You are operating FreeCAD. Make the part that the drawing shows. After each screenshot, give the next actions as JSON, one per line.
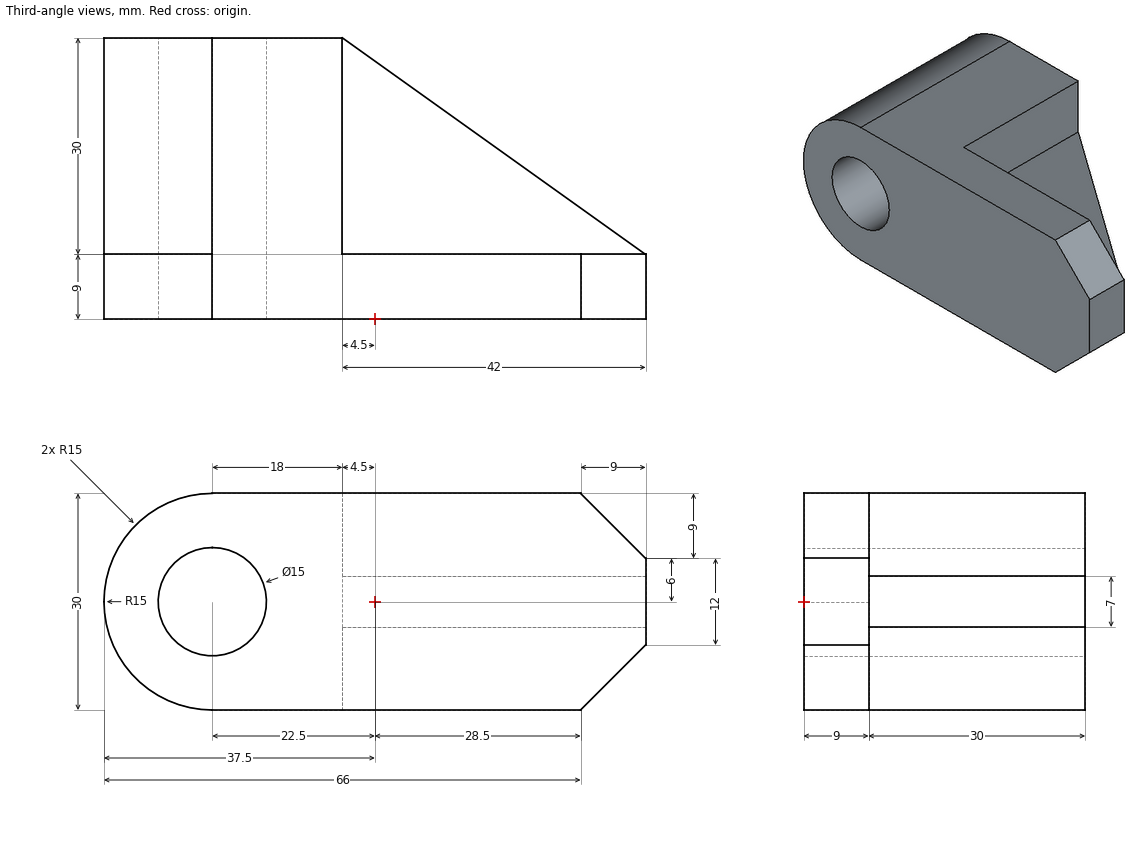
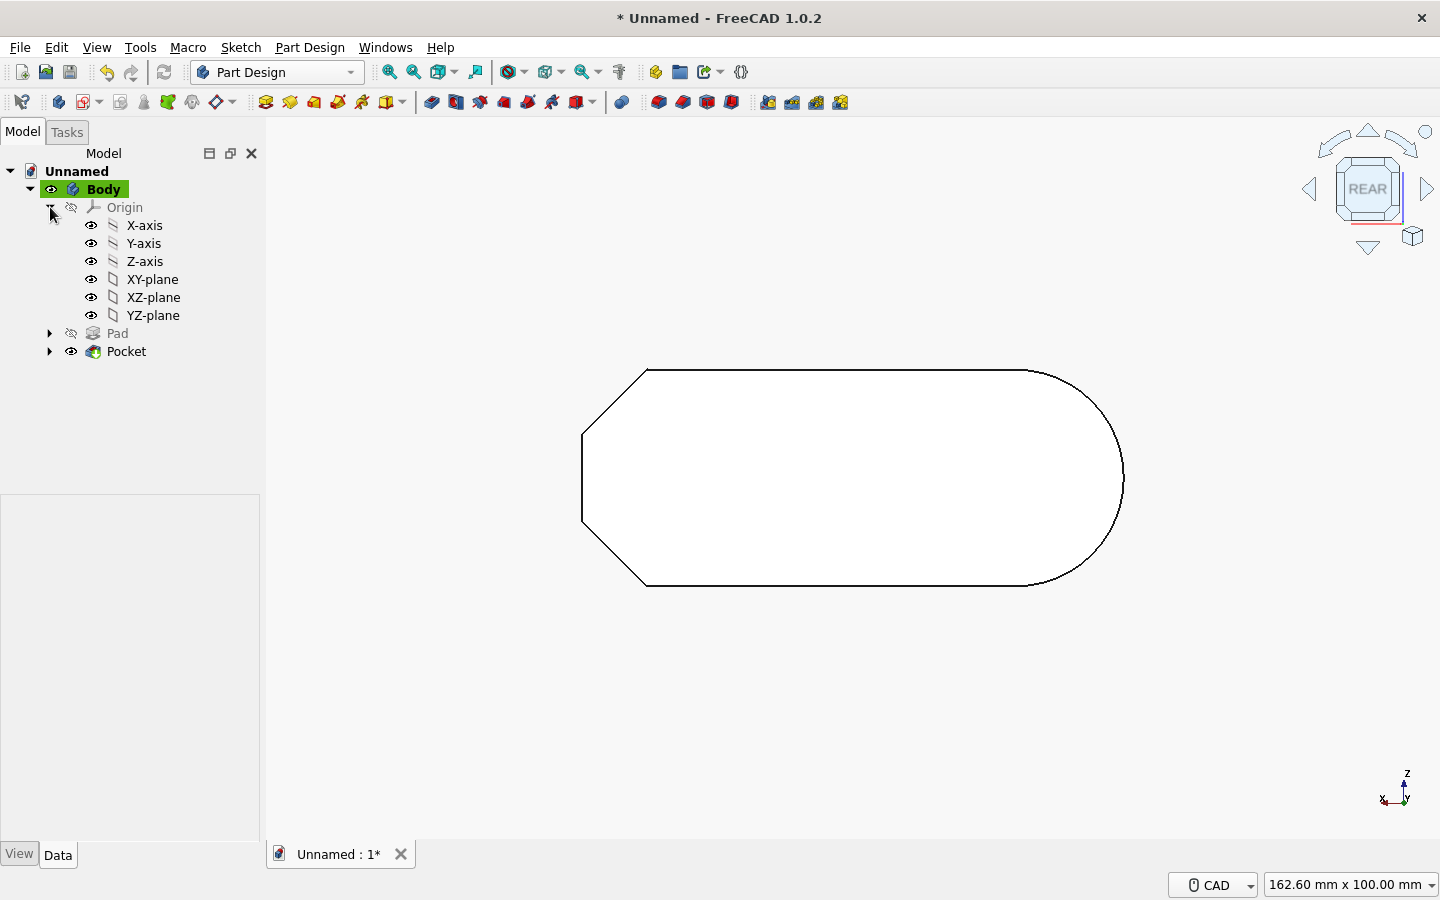
{"action": "left_click", "coordinate": [136, 297]}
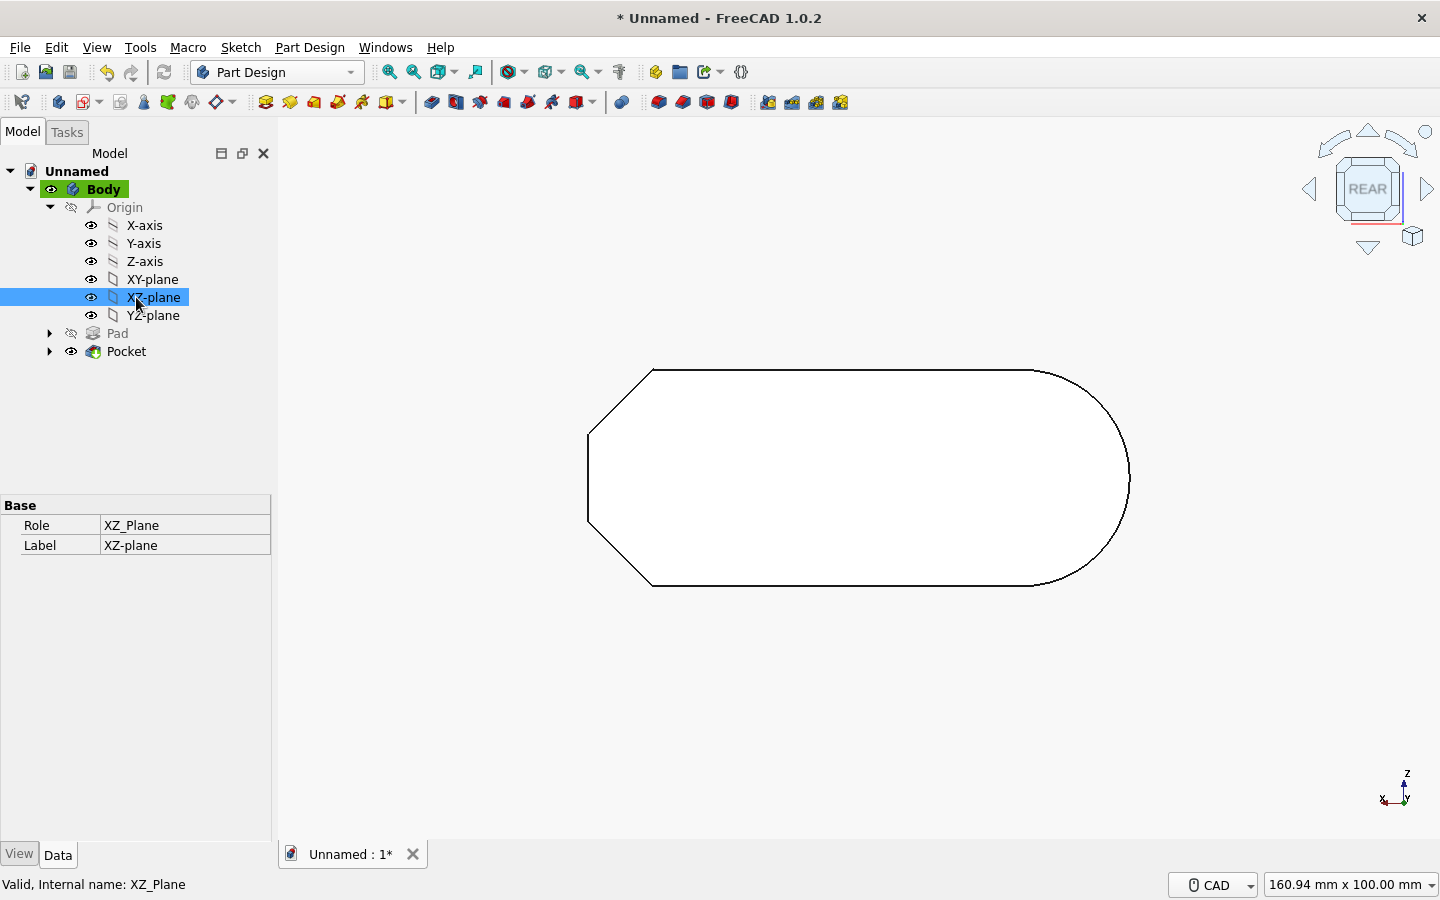
{"action": "left_click", "coordinate": [216, 102]}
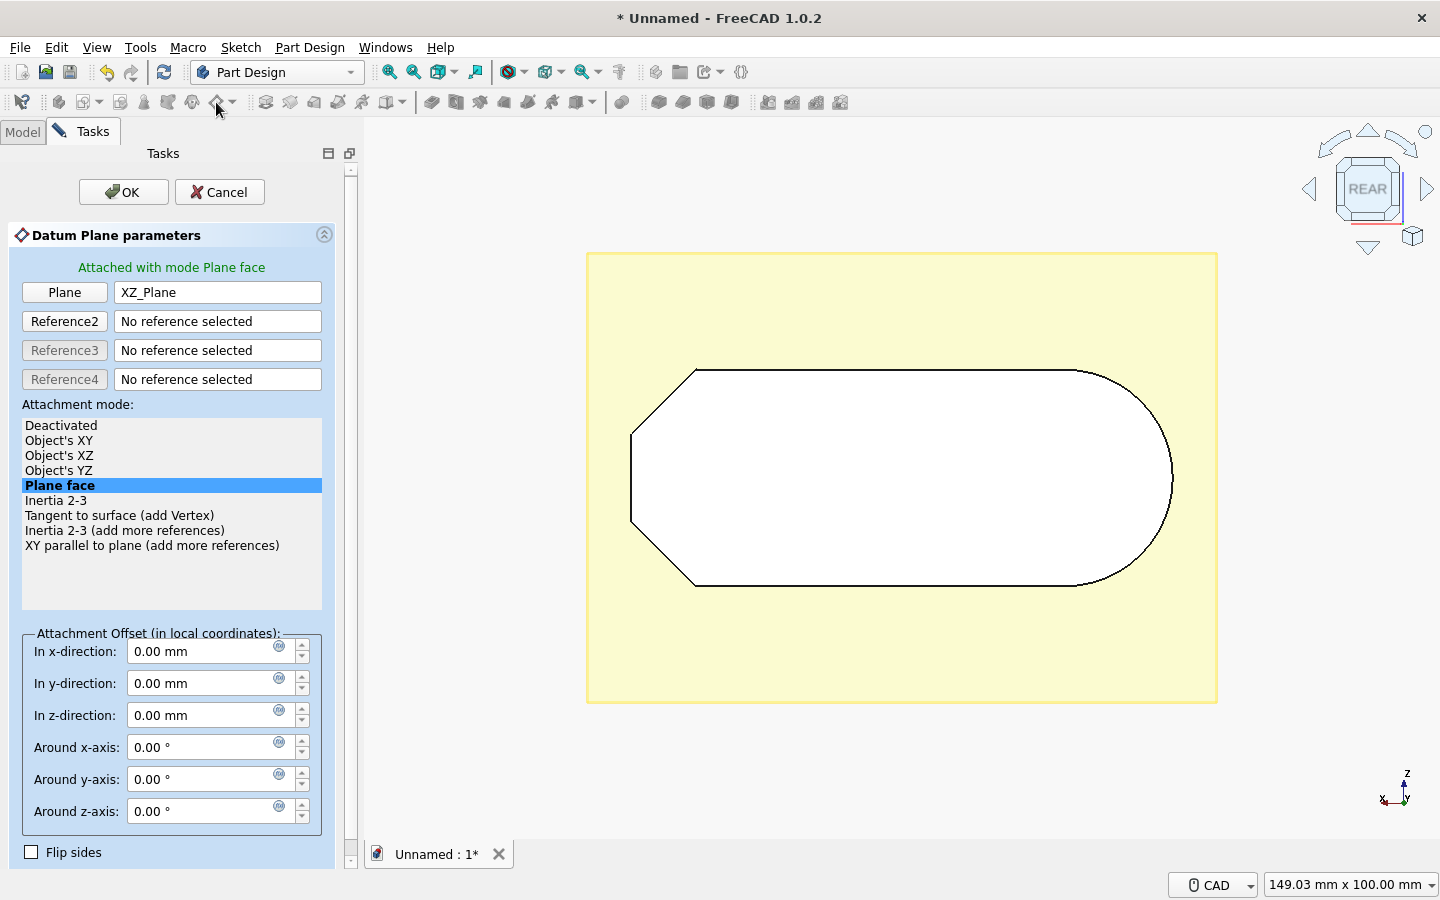
{"action": "triple_click", "coordinate": [210, 715]}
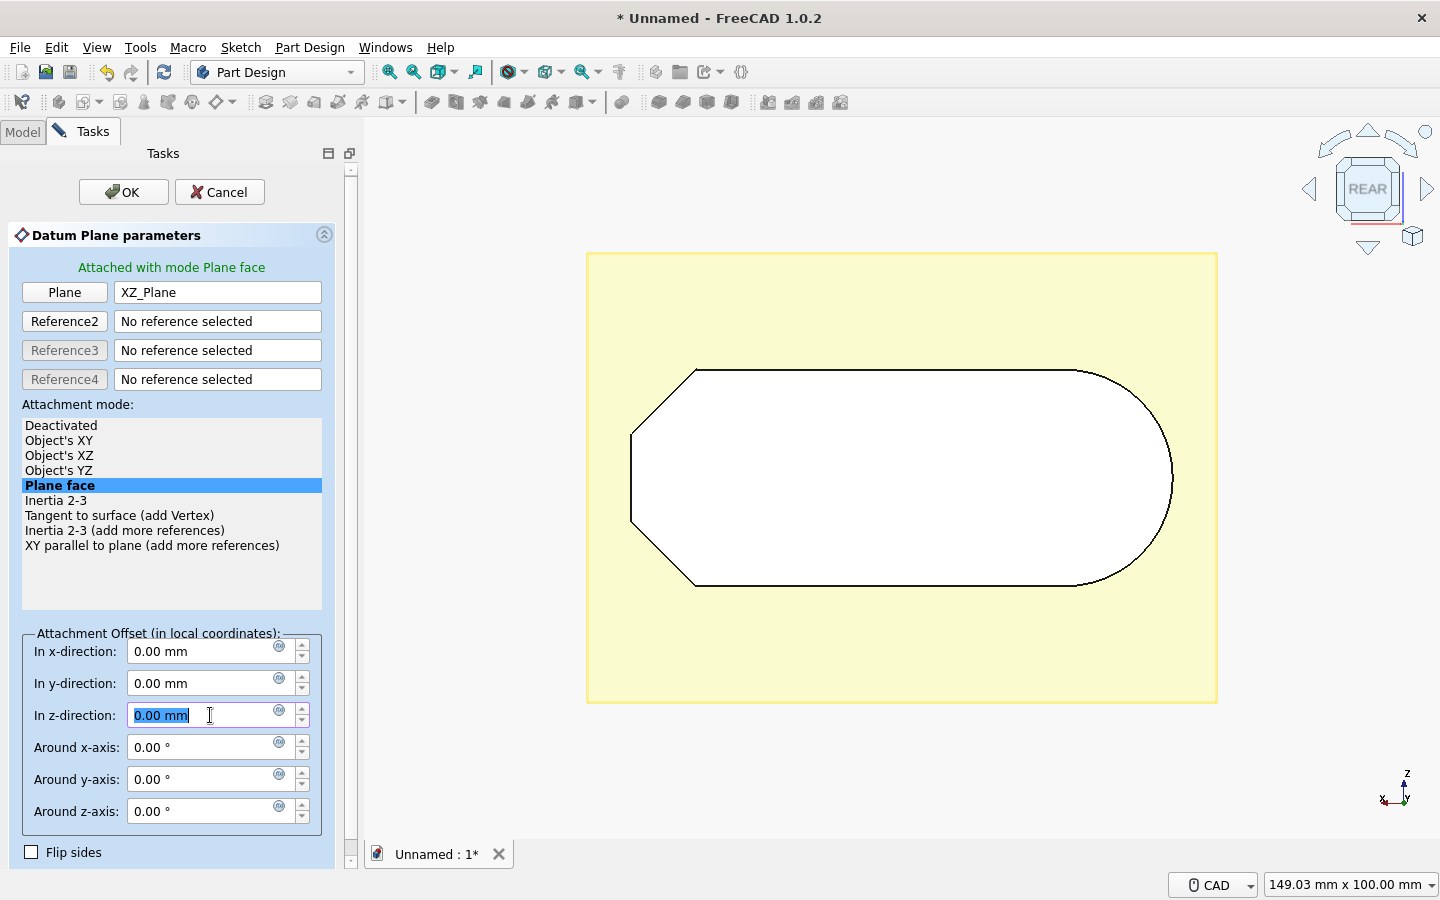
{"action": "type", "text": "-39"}
{"action": "key", "text": "Tab"}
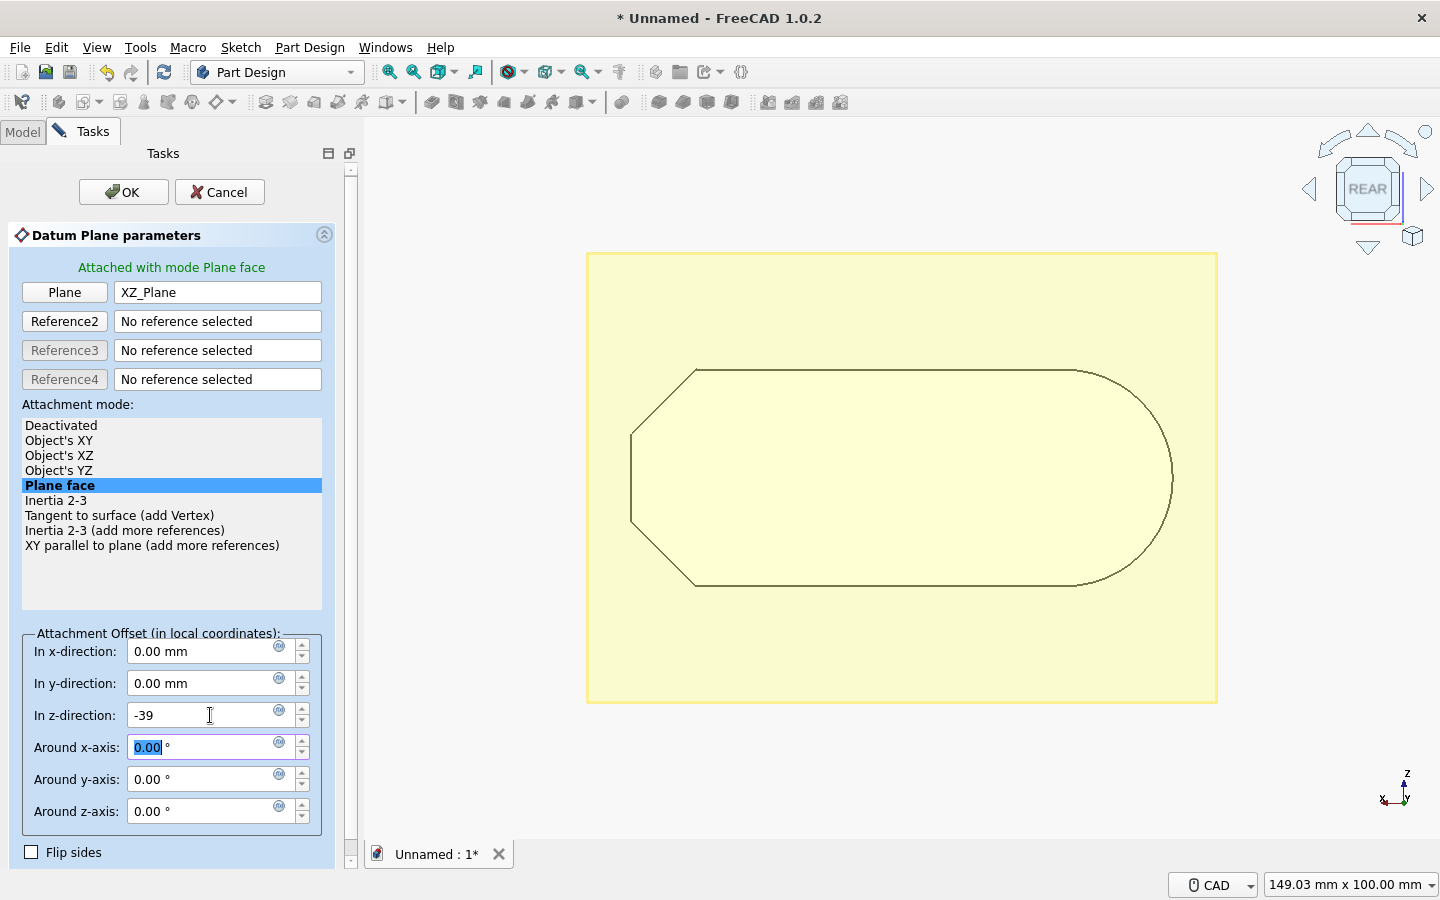
{"action": "left_click", "coordinate": [124, 192]}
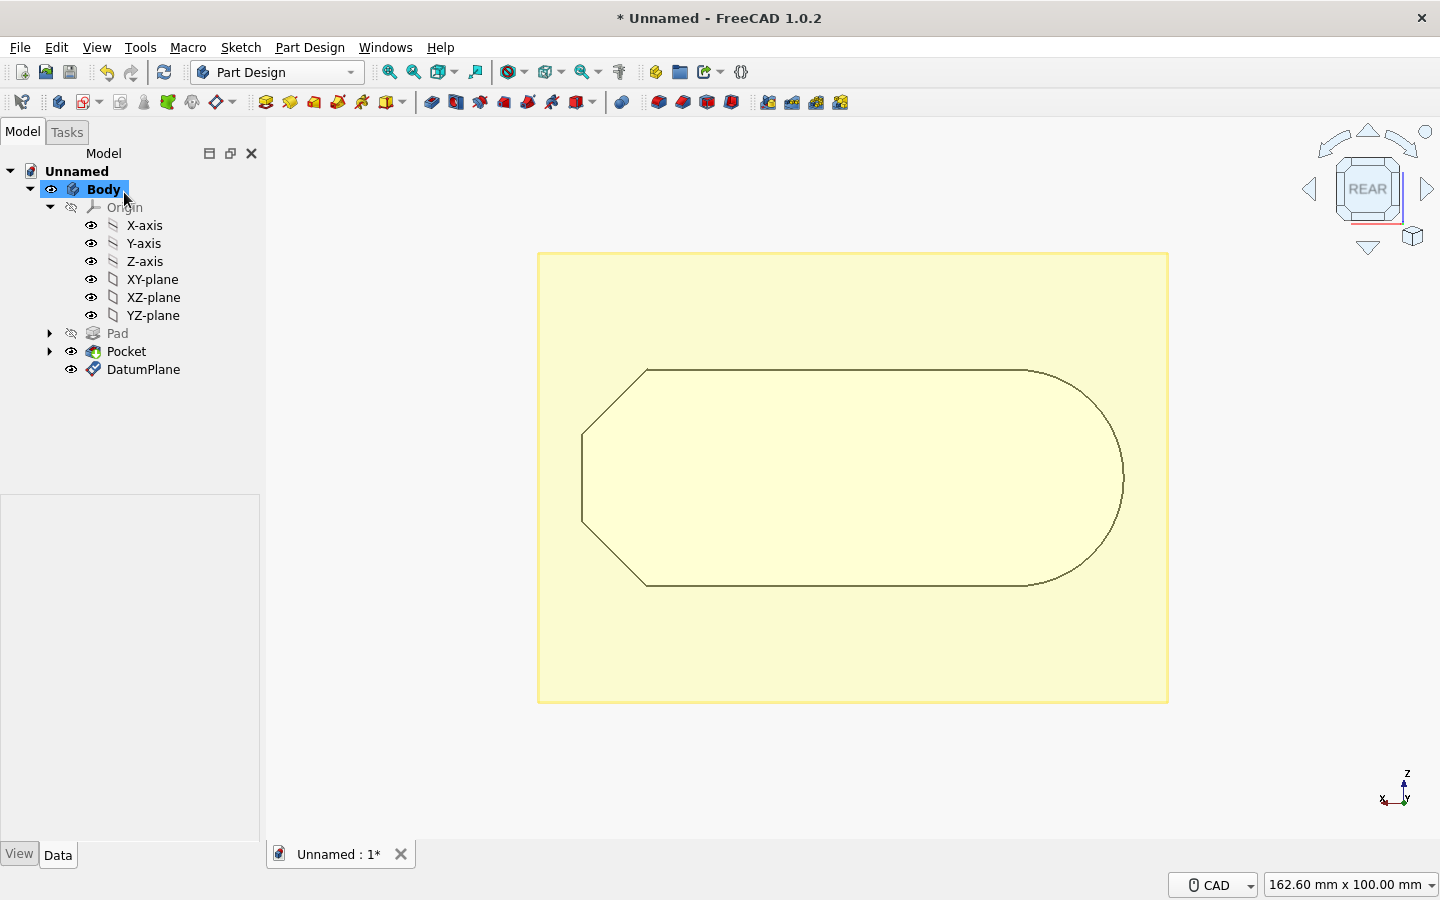
{"action": "left_click", "coordinate": [116, 369]}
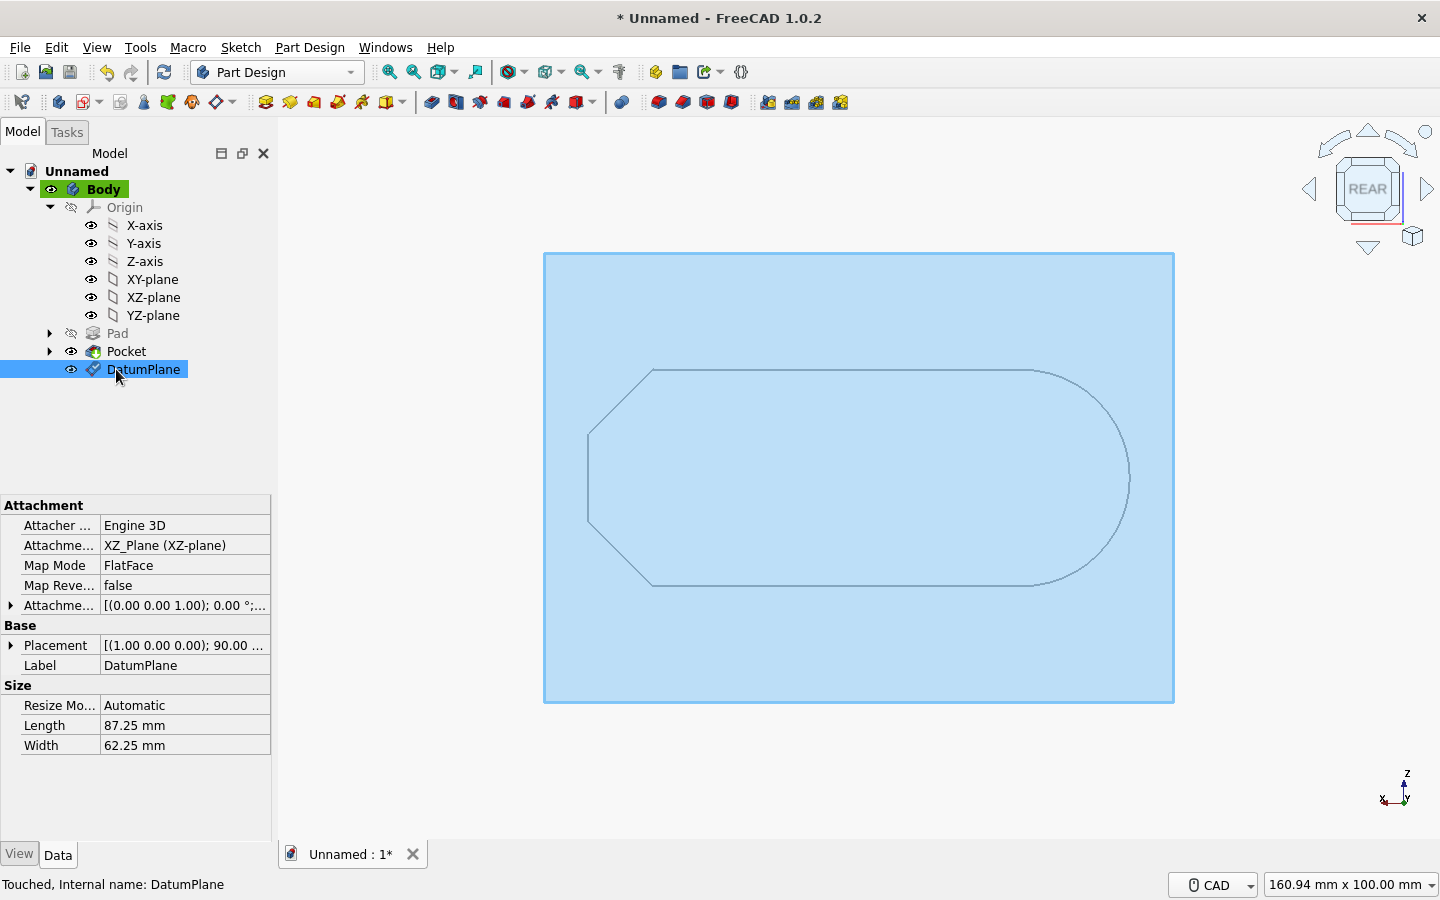
{"action": "left_click", "coordinate": [84, 102]}